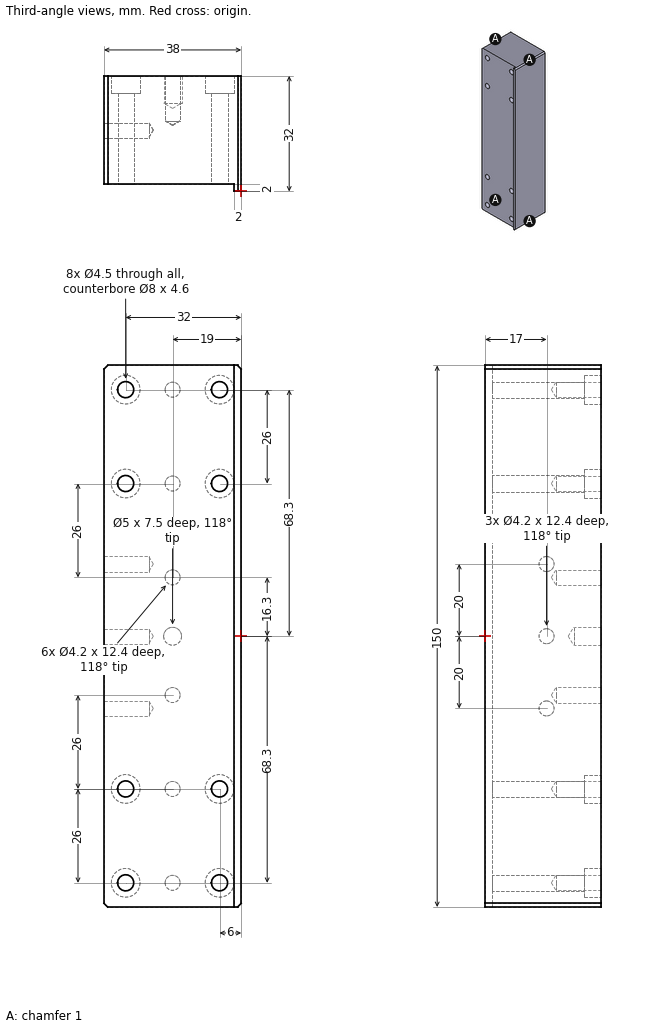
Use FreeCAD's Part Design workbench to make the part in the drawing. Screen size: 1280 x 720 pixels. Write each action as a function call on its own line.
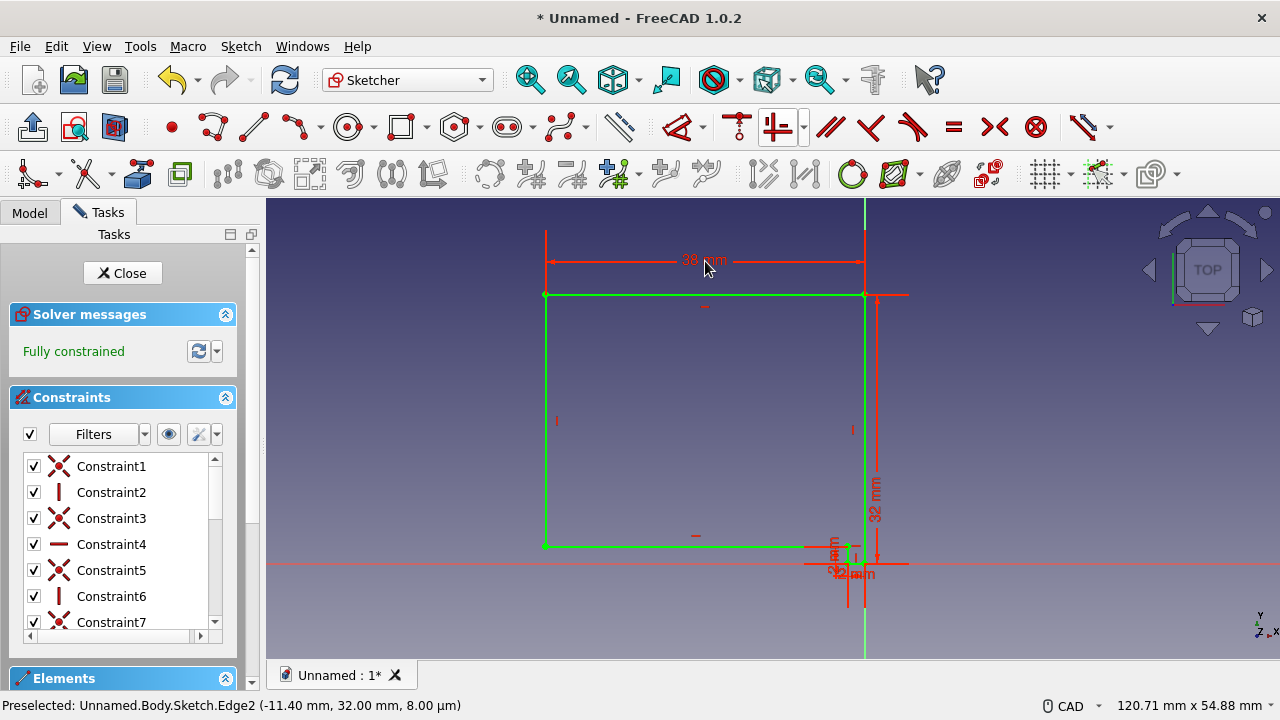
click(123, 273)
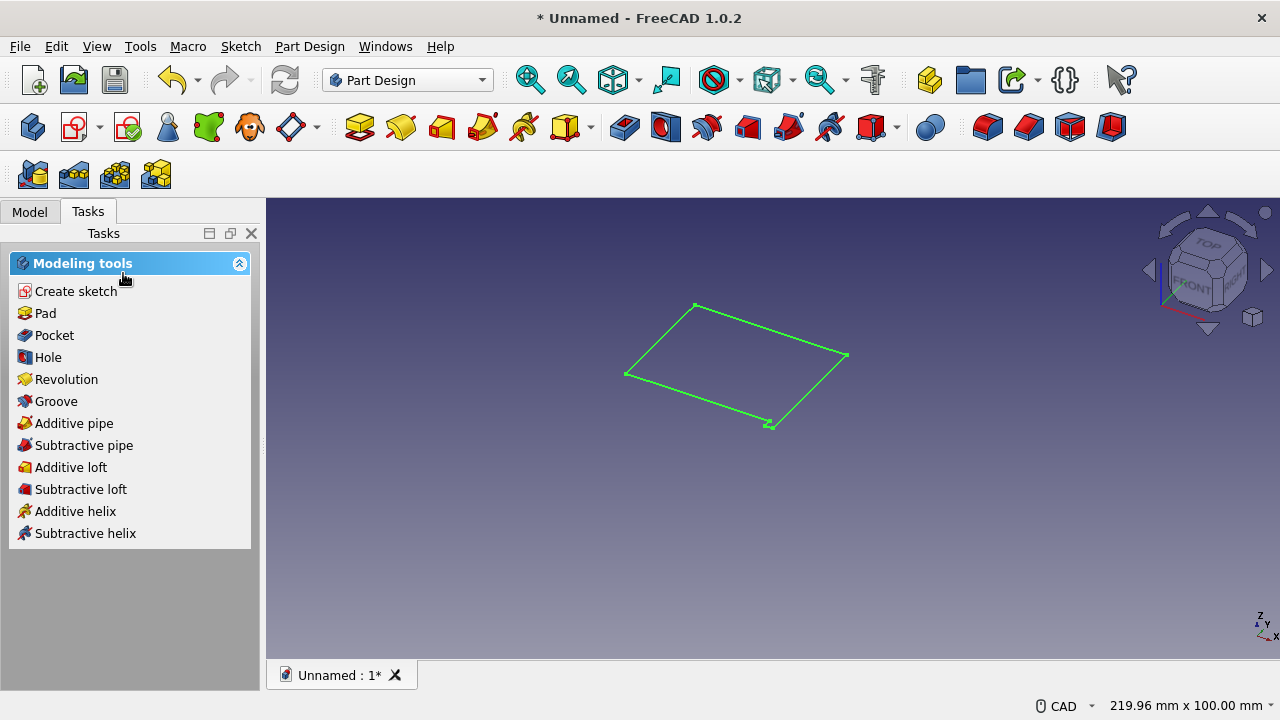
click(360, 128)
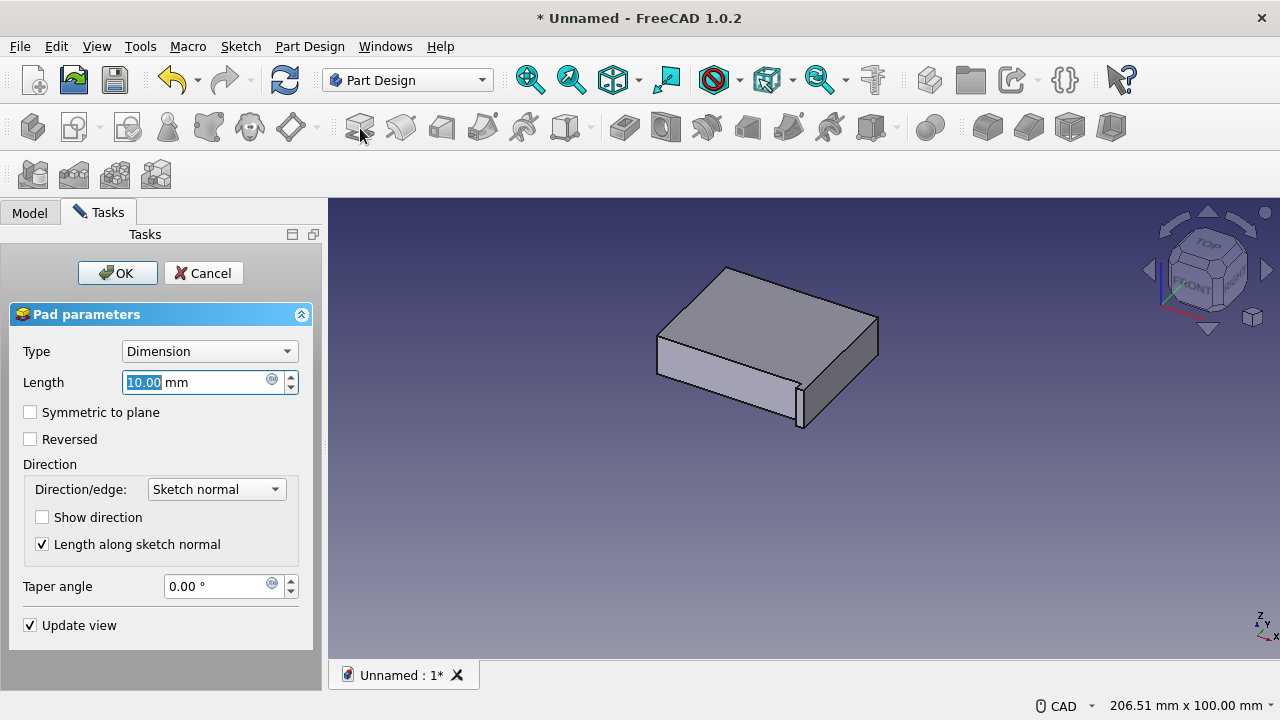
text(150)
key(Tab)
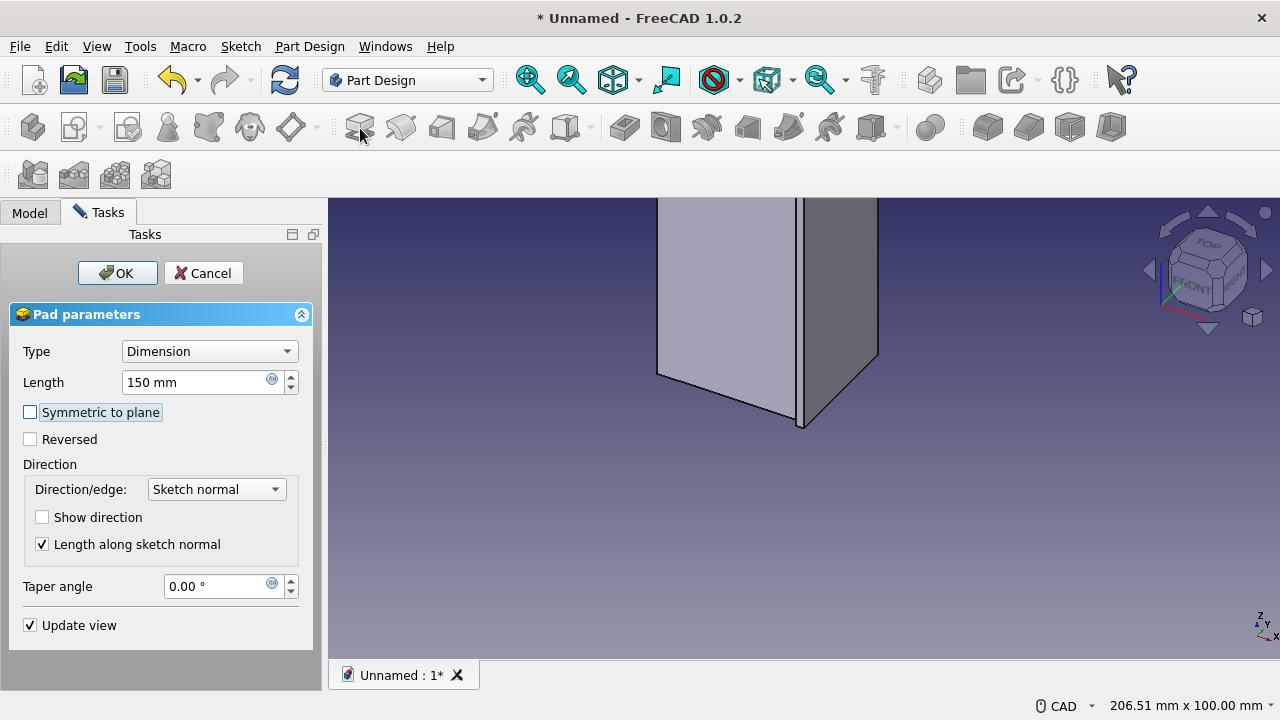
click(31, 412)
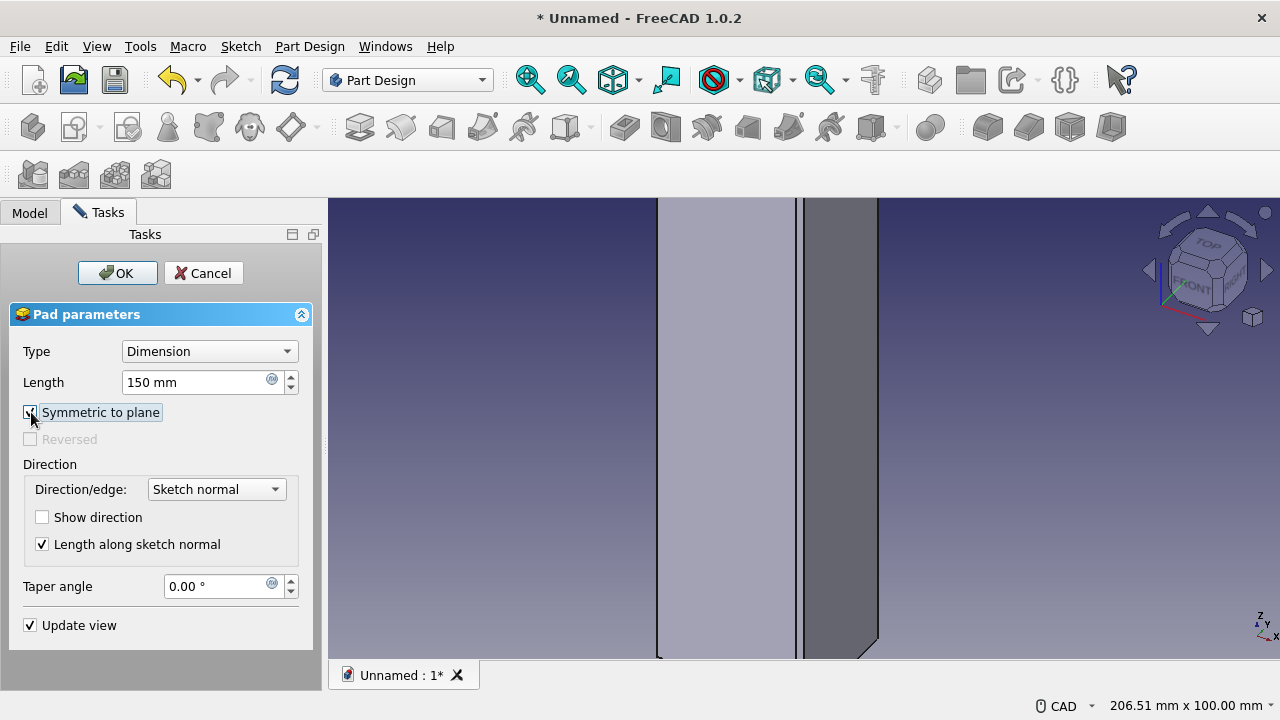
click(118, 273)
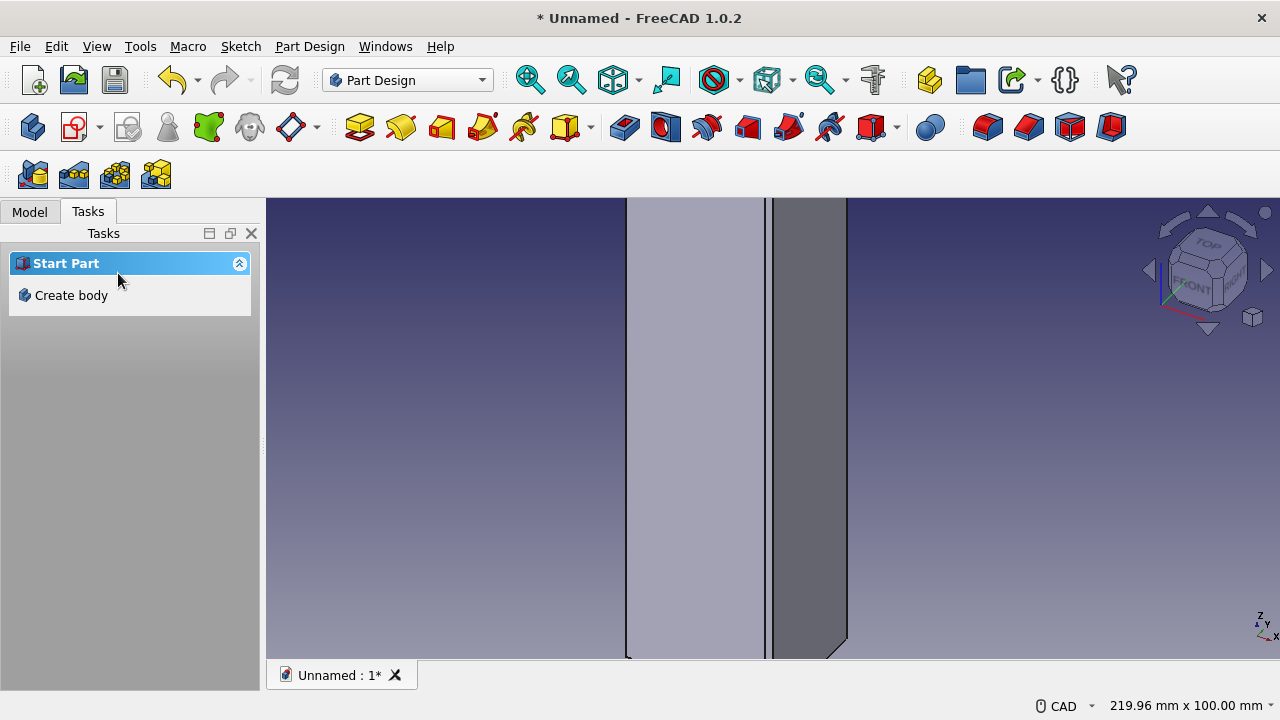
click(531, 80)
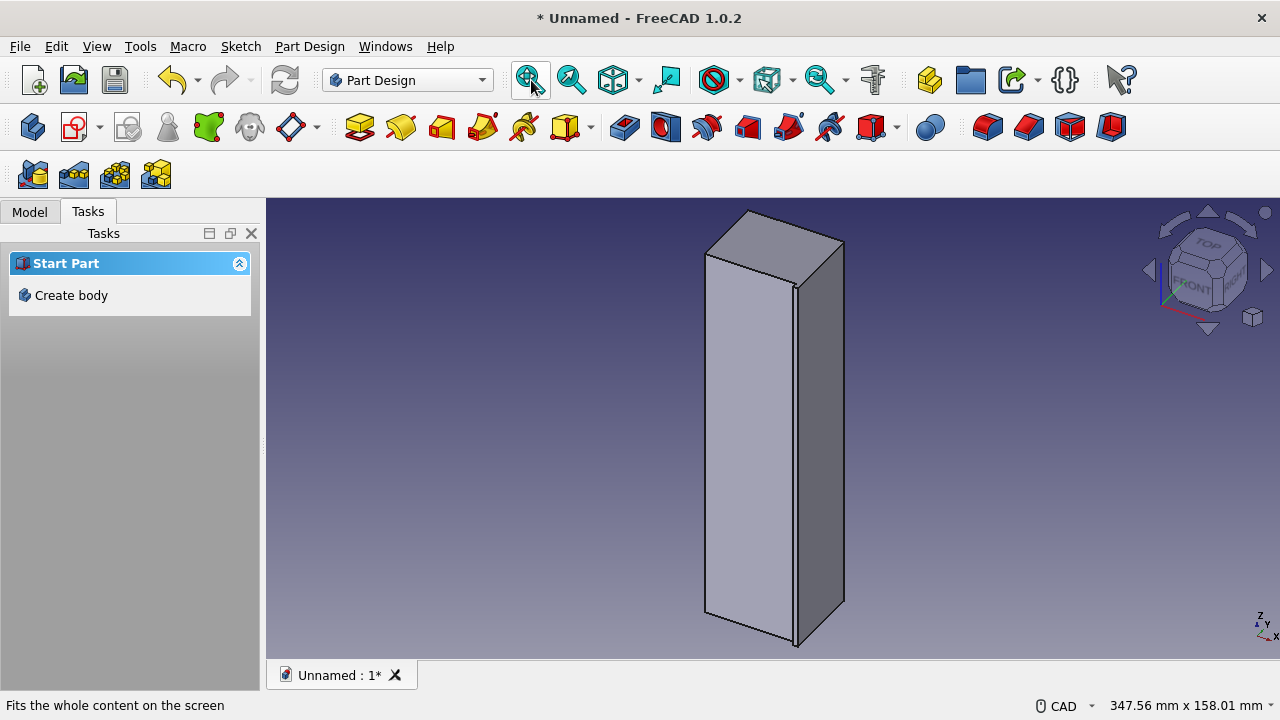
key(4)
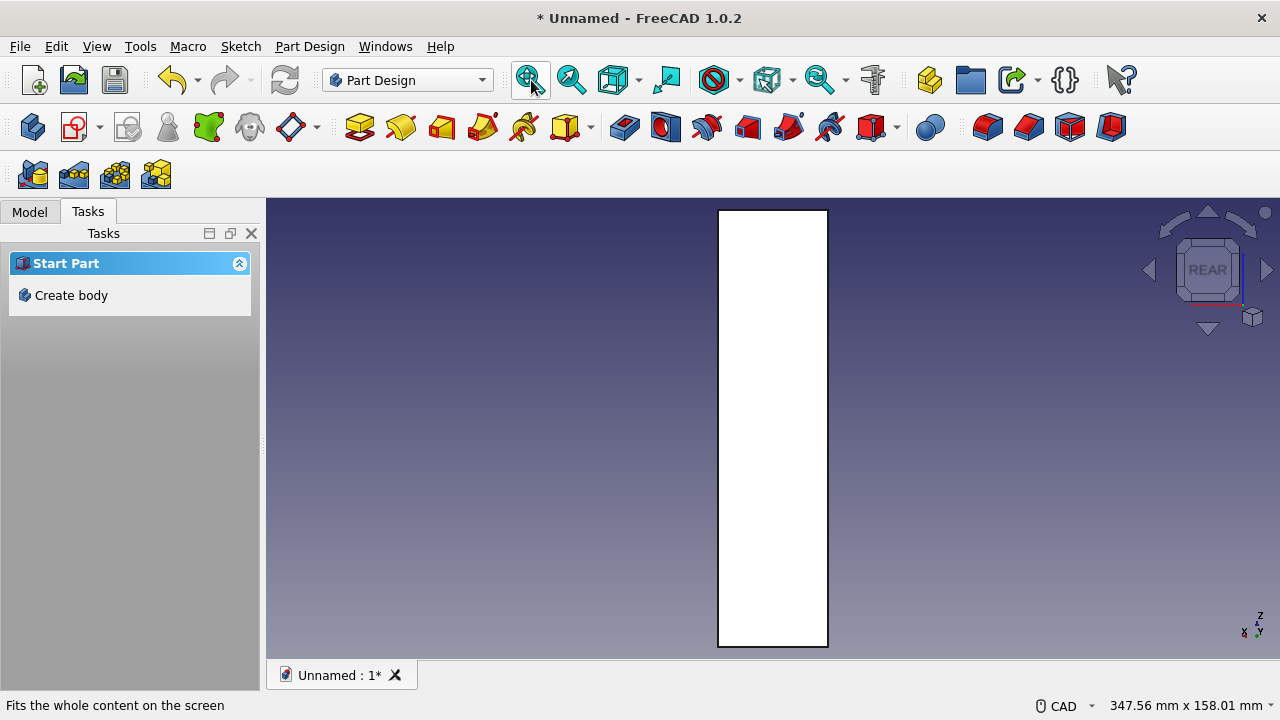
click(773, 302)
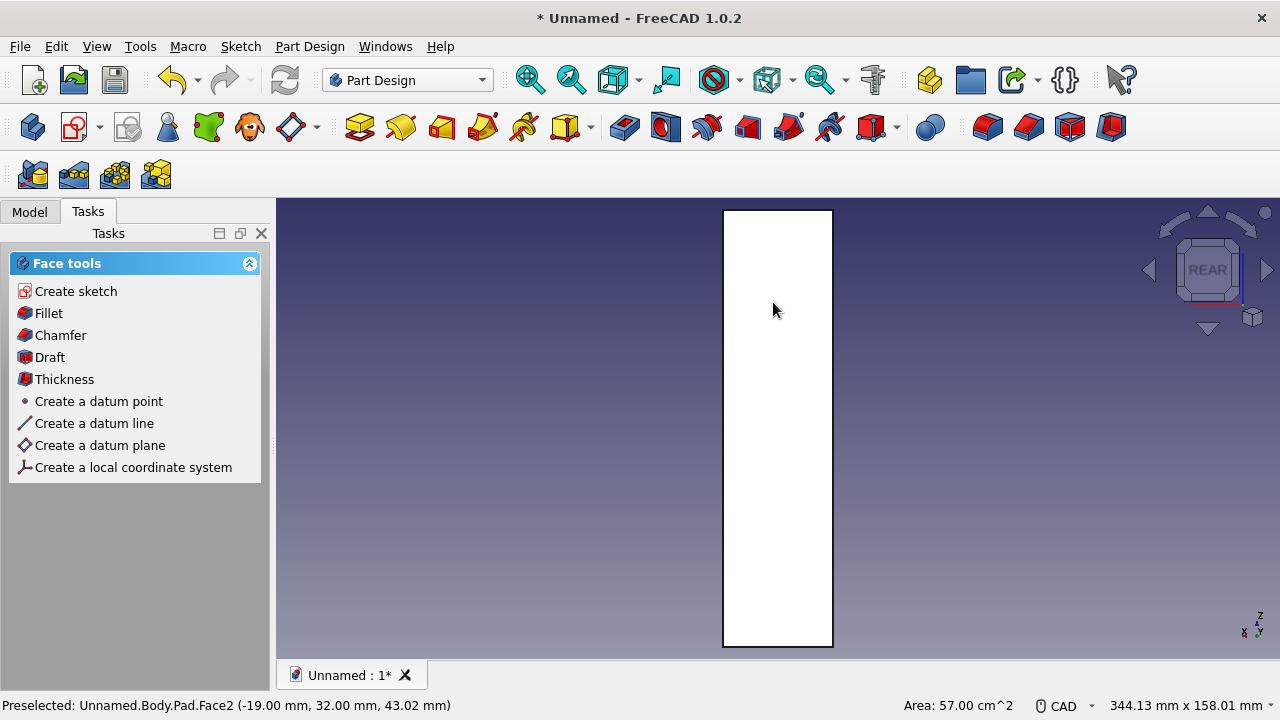
click(74, 128)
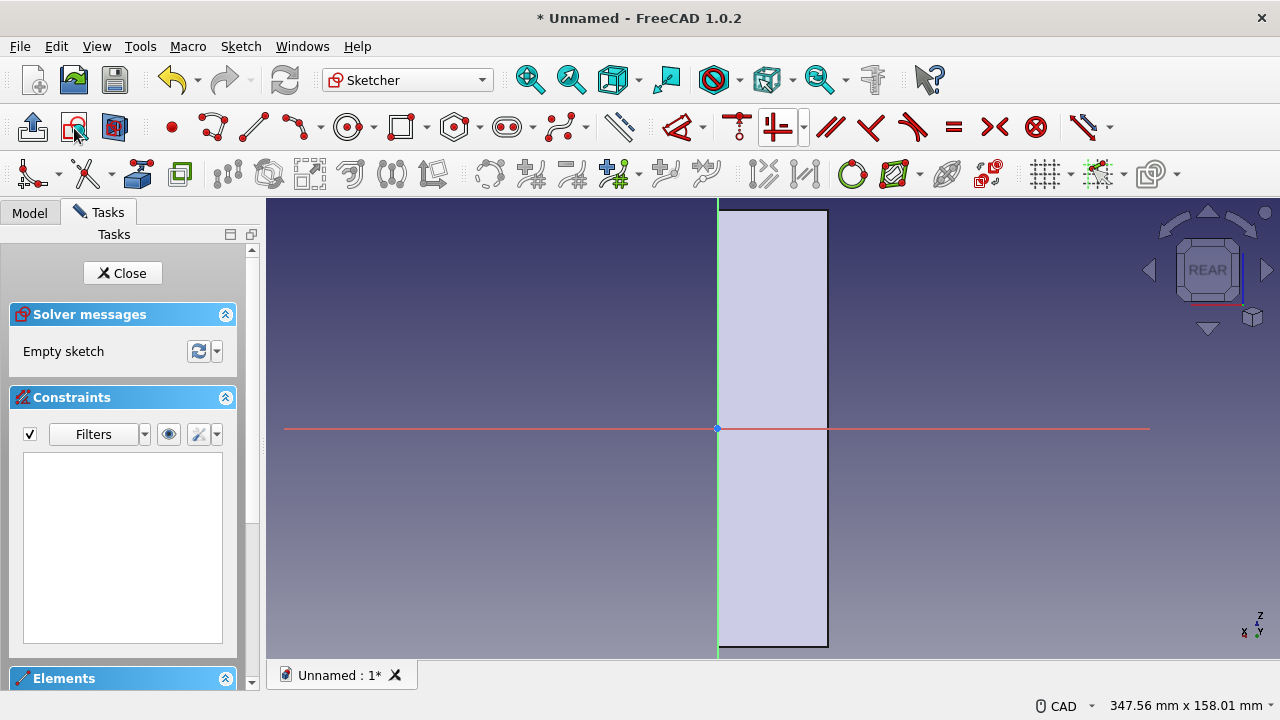
scroll(576, 429, down, 2)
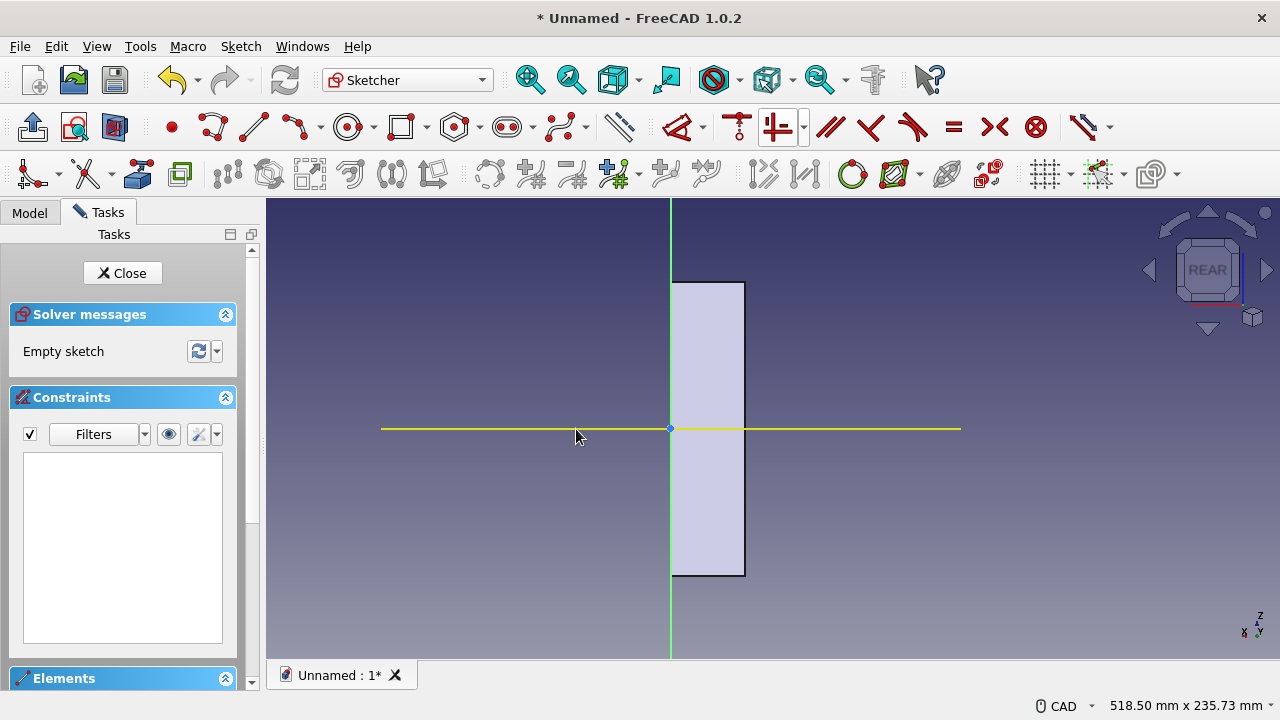
click(348, 128)